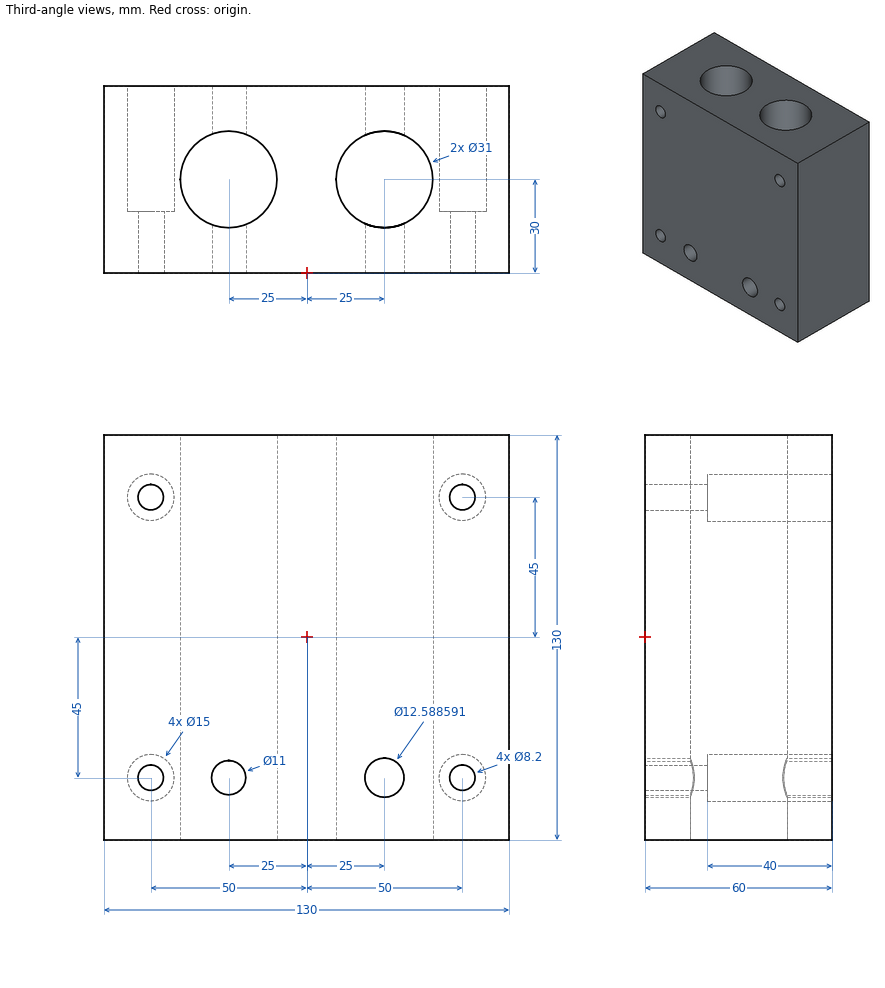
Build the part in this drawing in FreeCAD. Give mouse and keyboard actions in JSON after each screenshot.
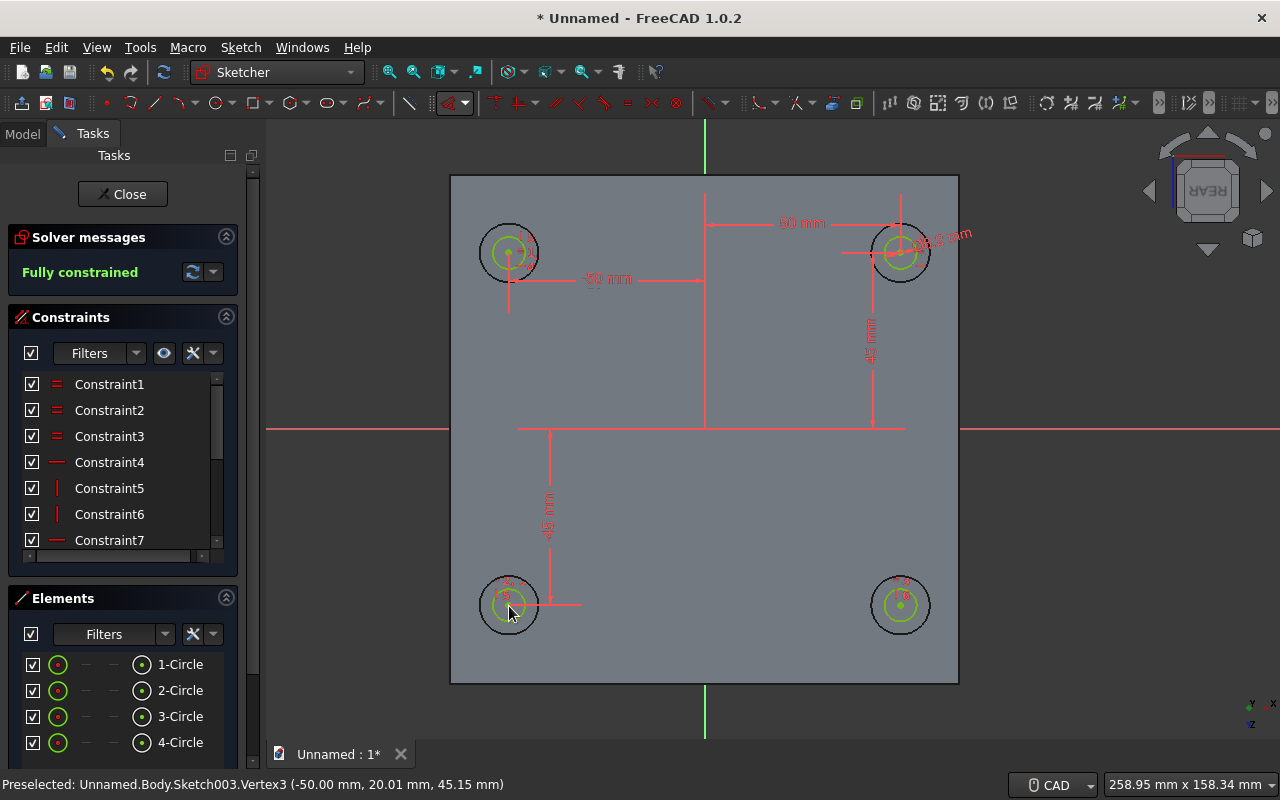
{"action": "left_click", "coordinate": [123, 194]}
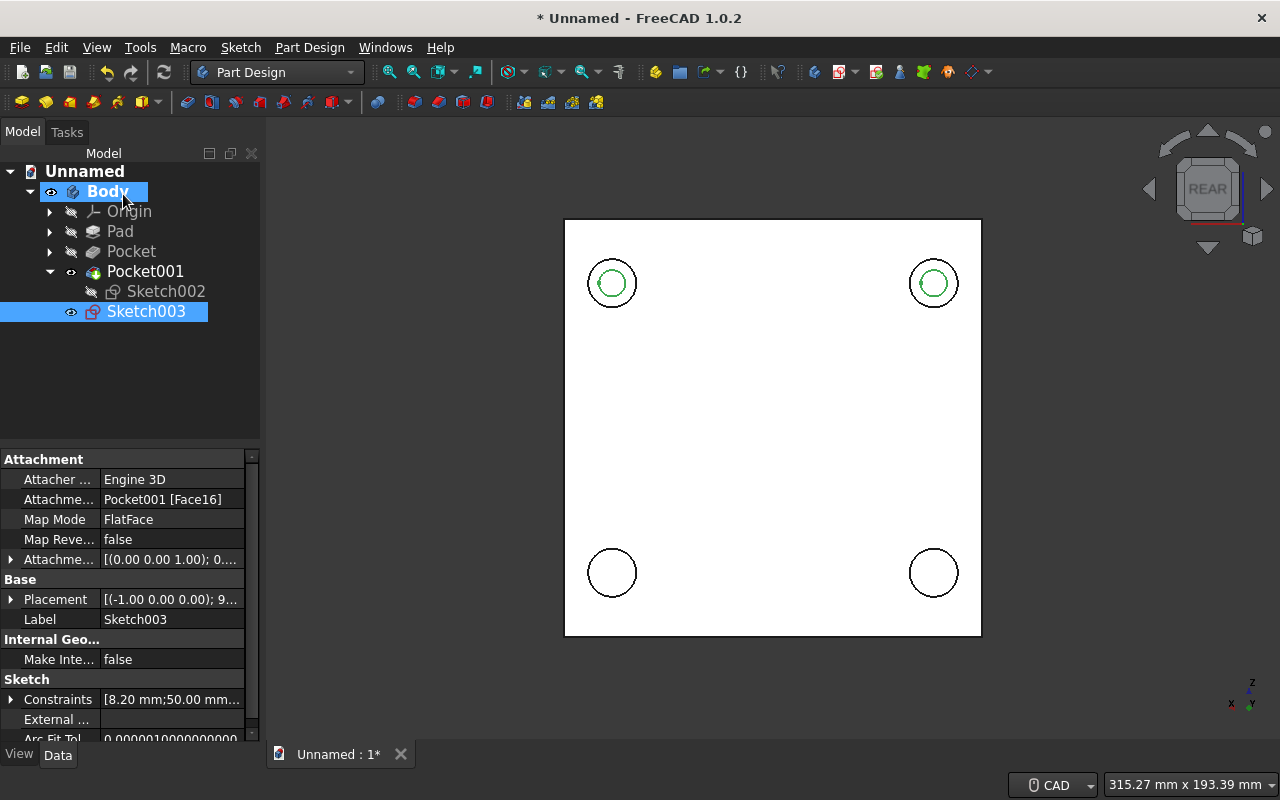
{"action": "left_click", "coordinate": [188, 102]}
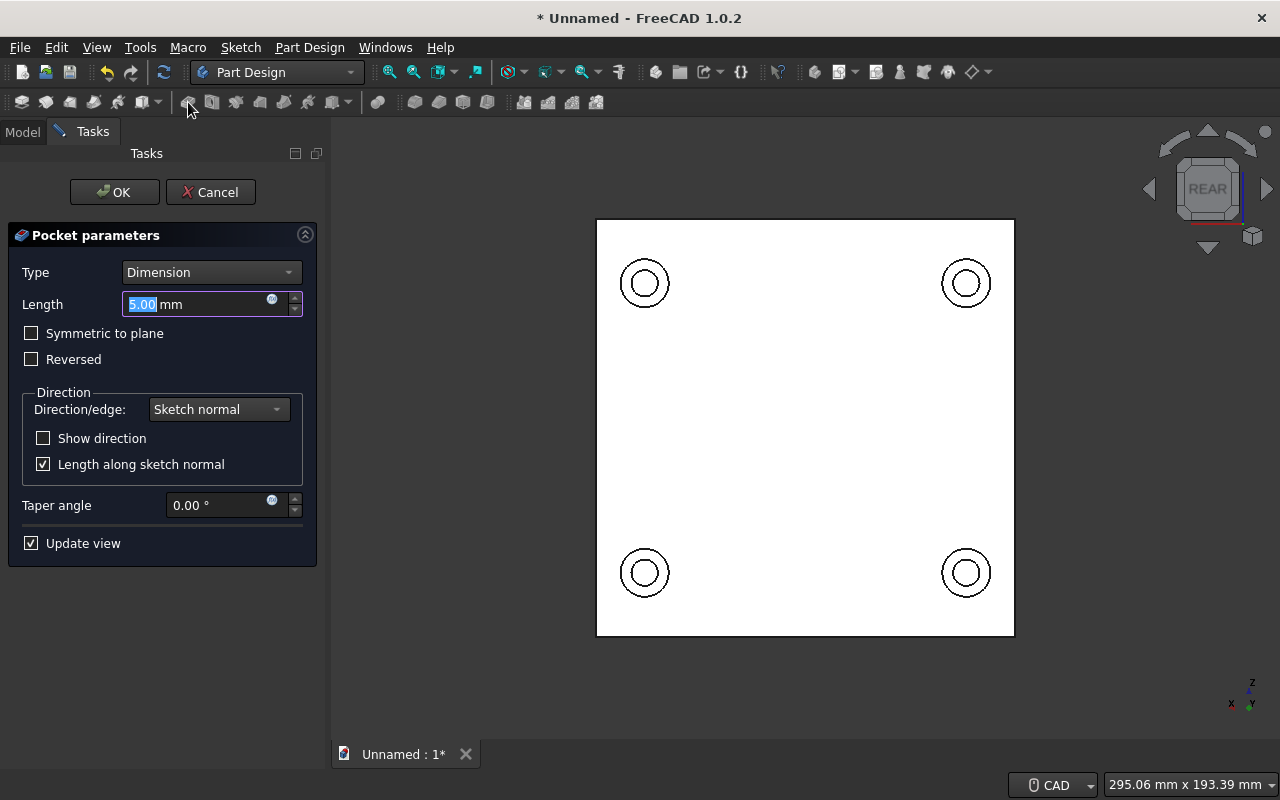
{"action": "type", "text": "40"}
{"action": "key", "text": "Tab"}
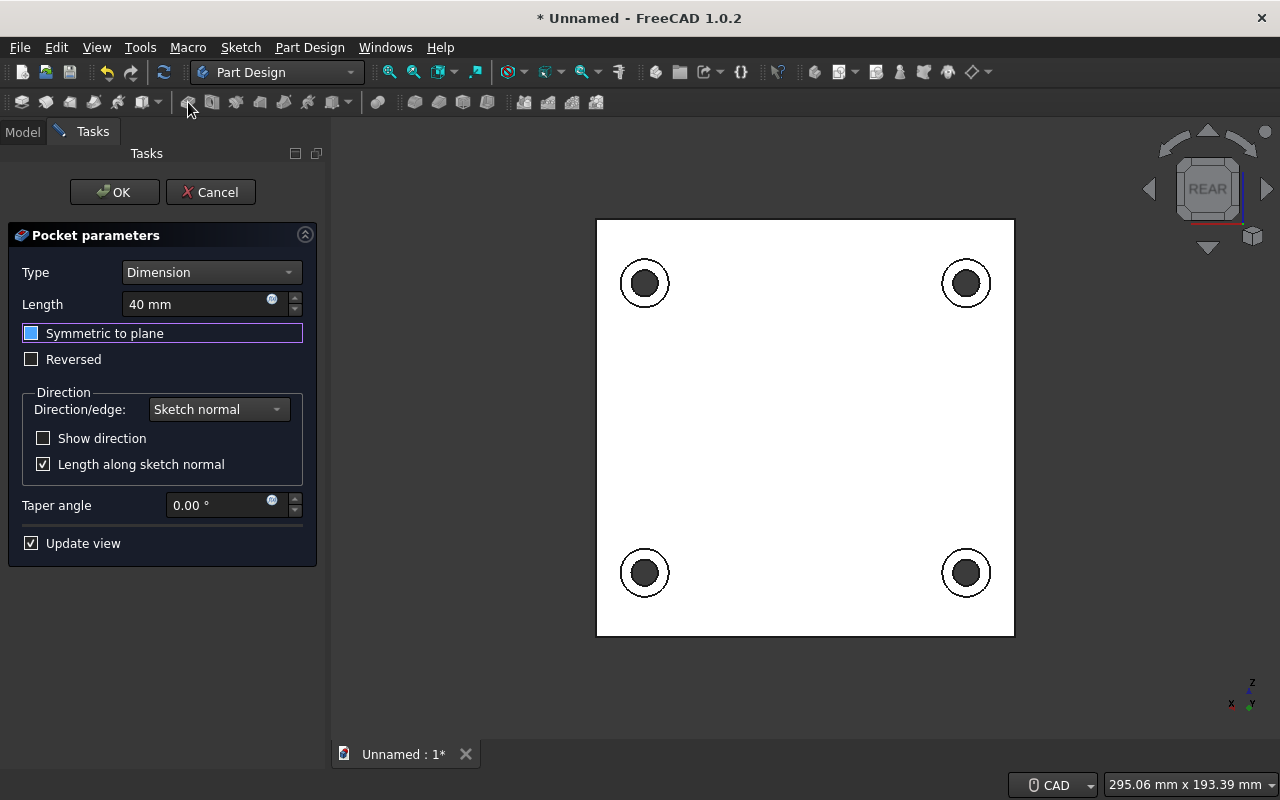
{"action": "left_click", "coordinate": [115, 192]}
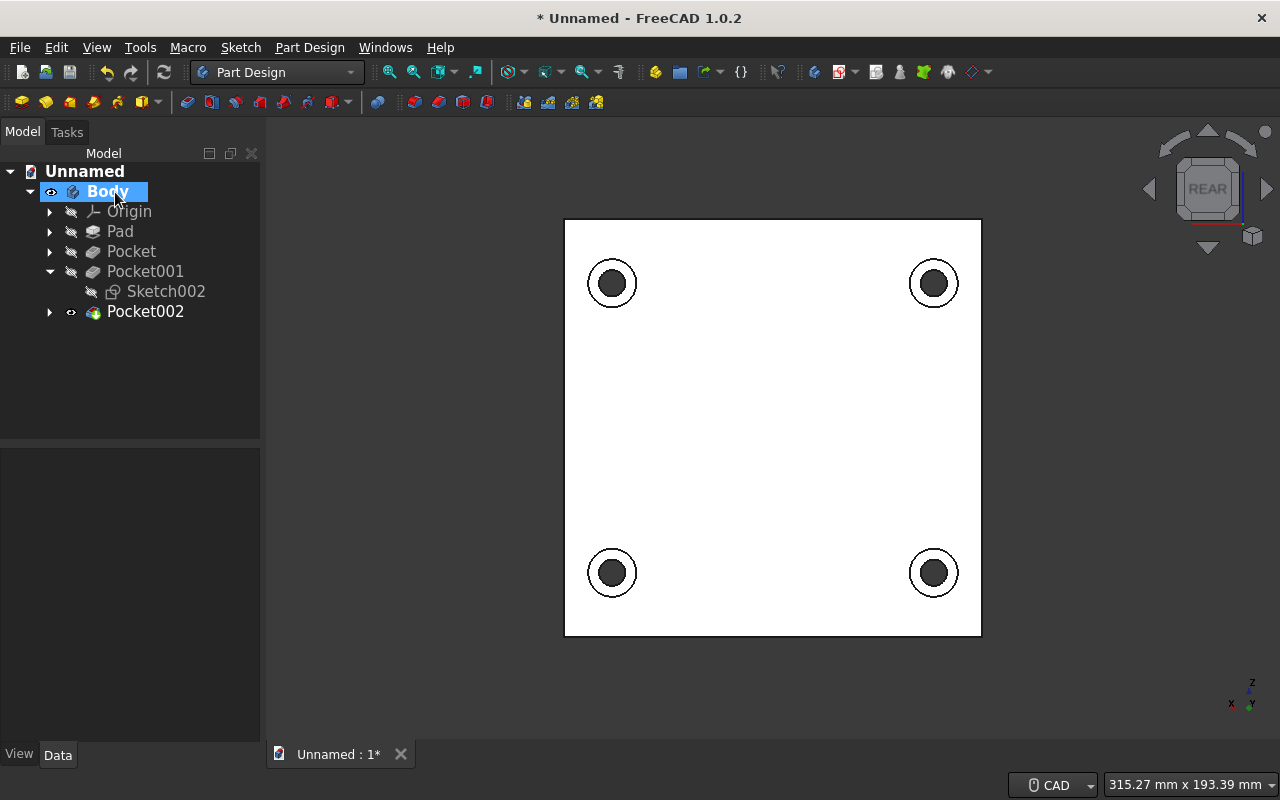
{"action": "left_click", "coordinate": [773, 427]}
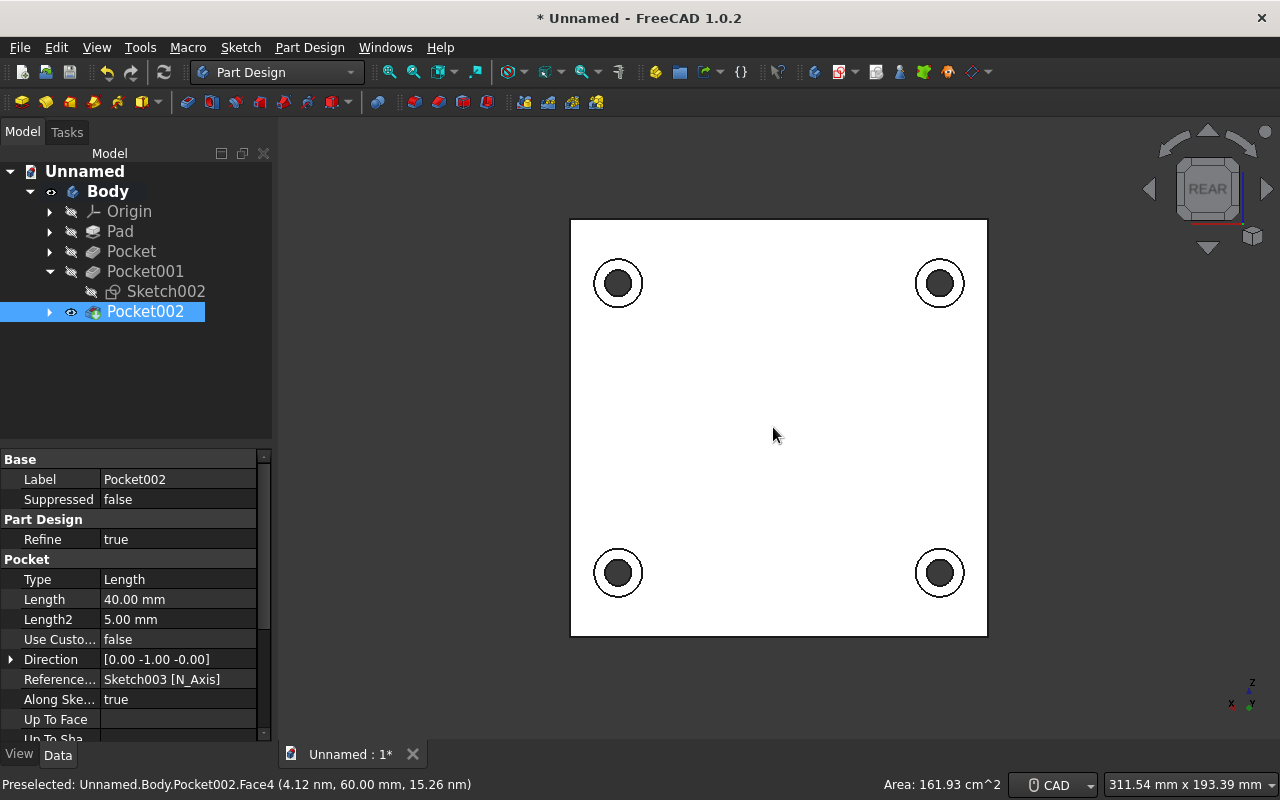
{"action": "left_click", "coordinate": [840, 72]}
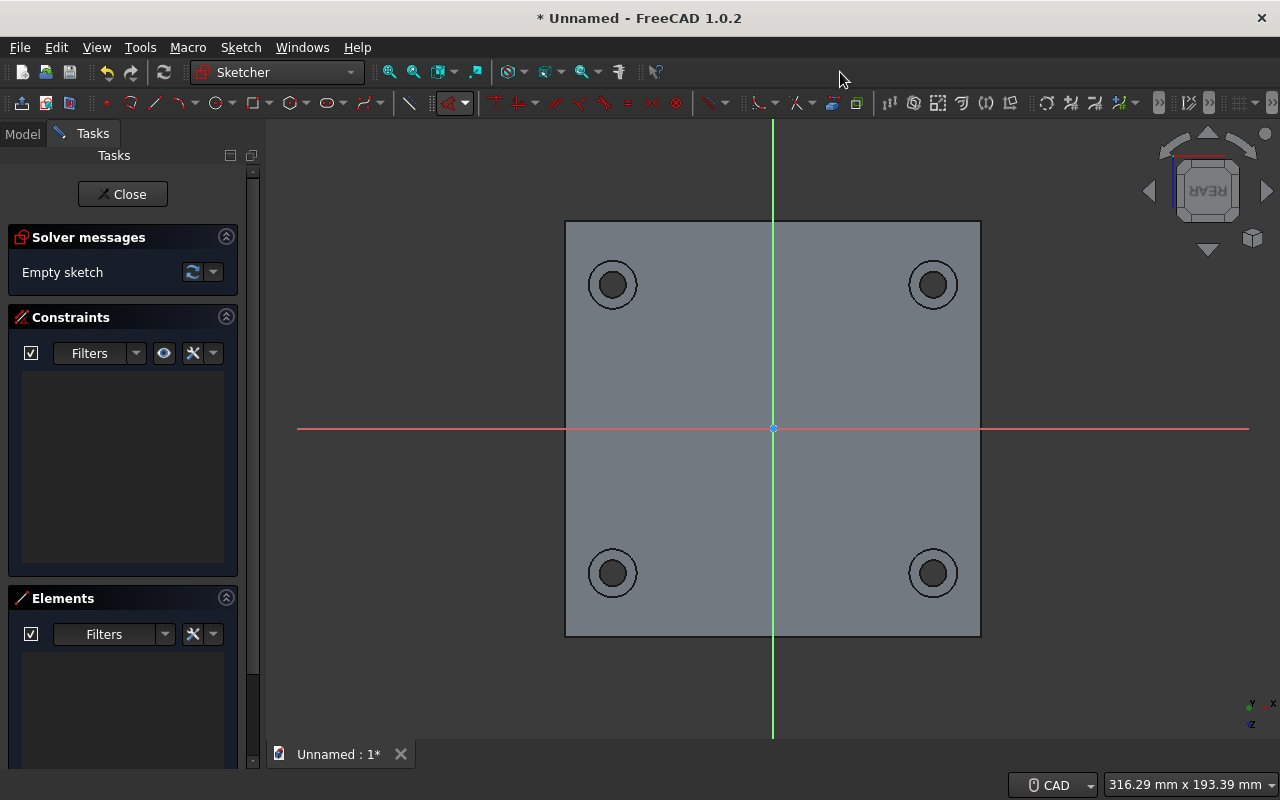
{"action": "scroll", "coordinate": [831, 280], "scroll_direction": "up", "scroll_amount": 4}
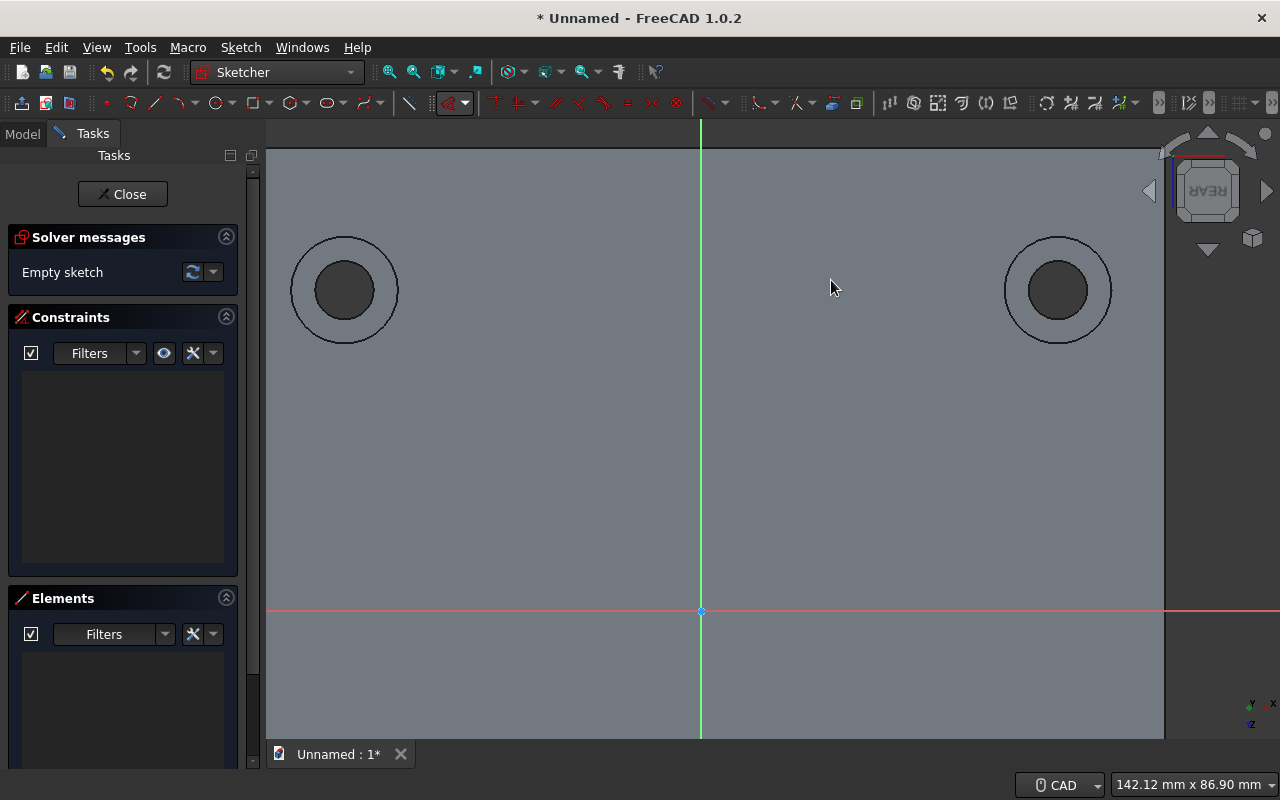
{"action": "key", "text": "g c"}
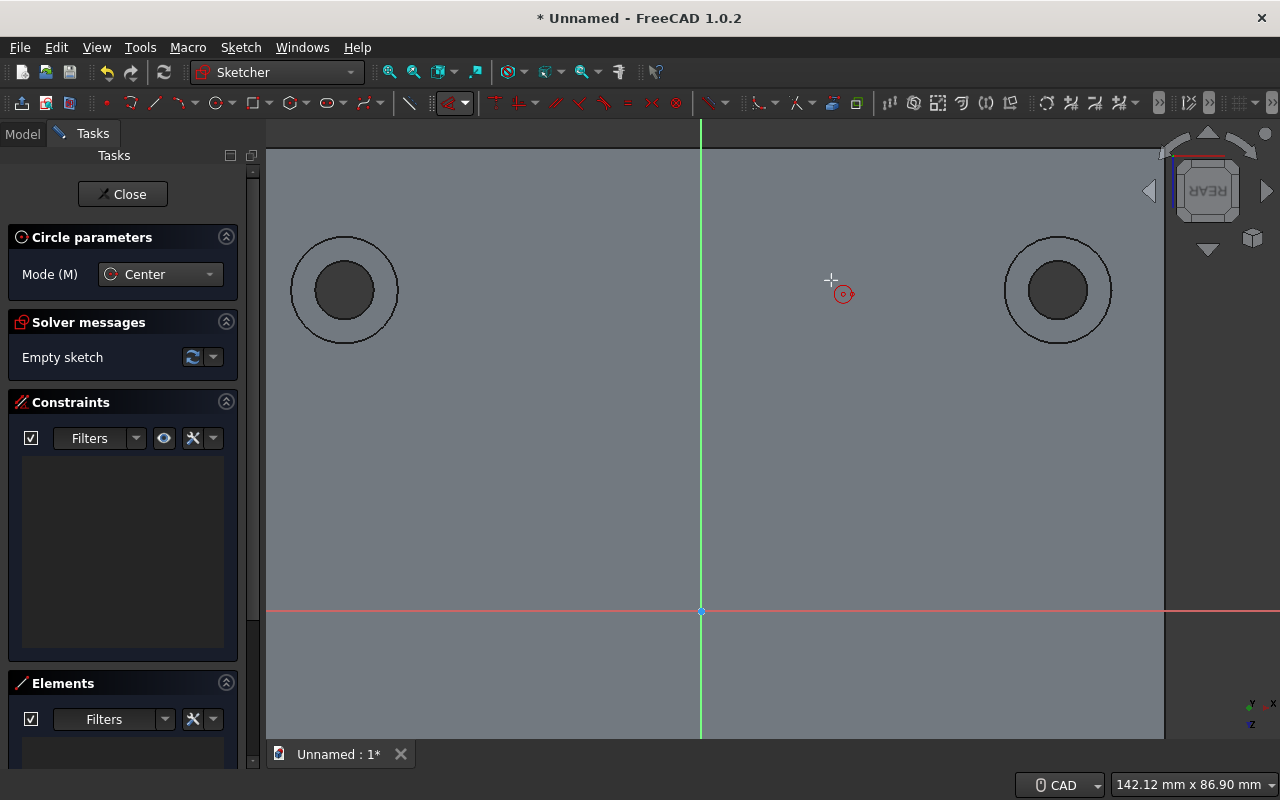
{"action": "left_click", "coordinate": [880, 290]}
{"action": "left_click", "coordinate": [911, 258]}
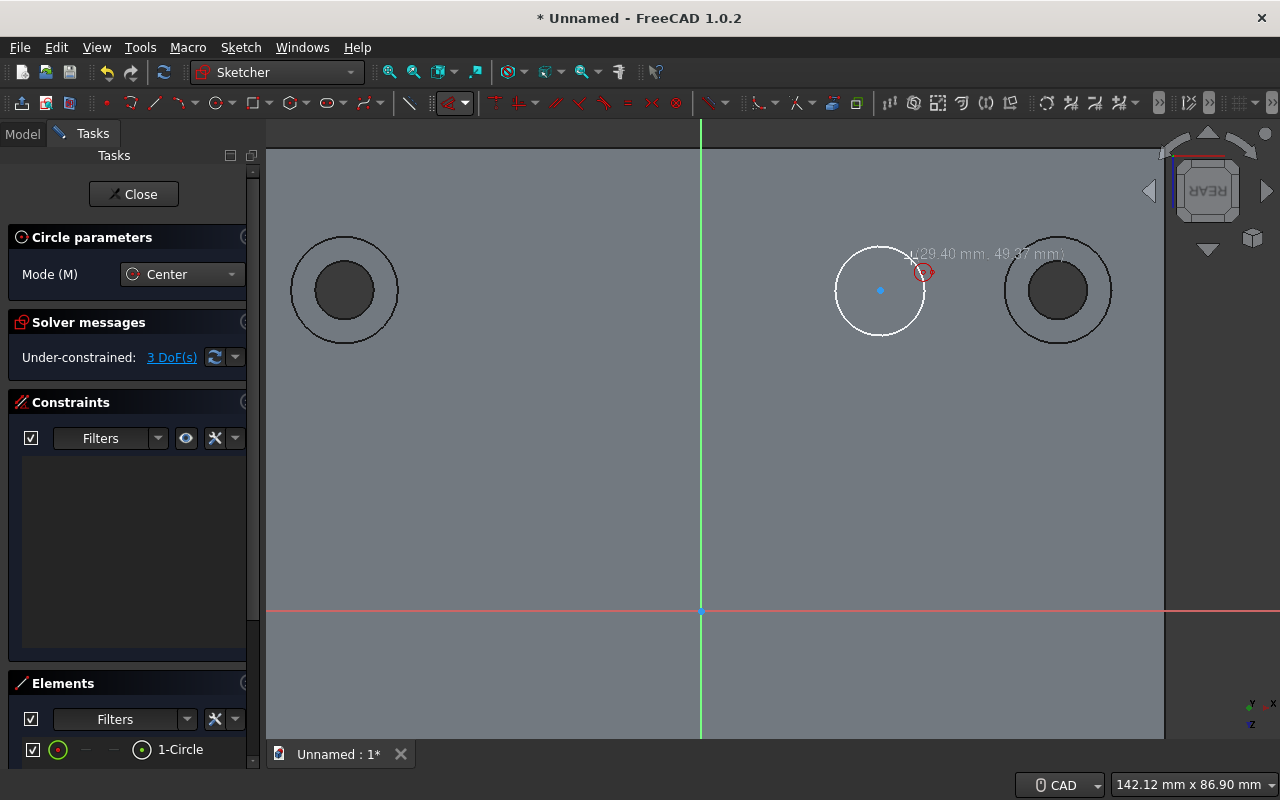
{"action": "left_click", "coordinate": [523, 290]}
{"action": "left_click", "coordinate": [551, 262]}
{"action": "key", "text": "Escape"}